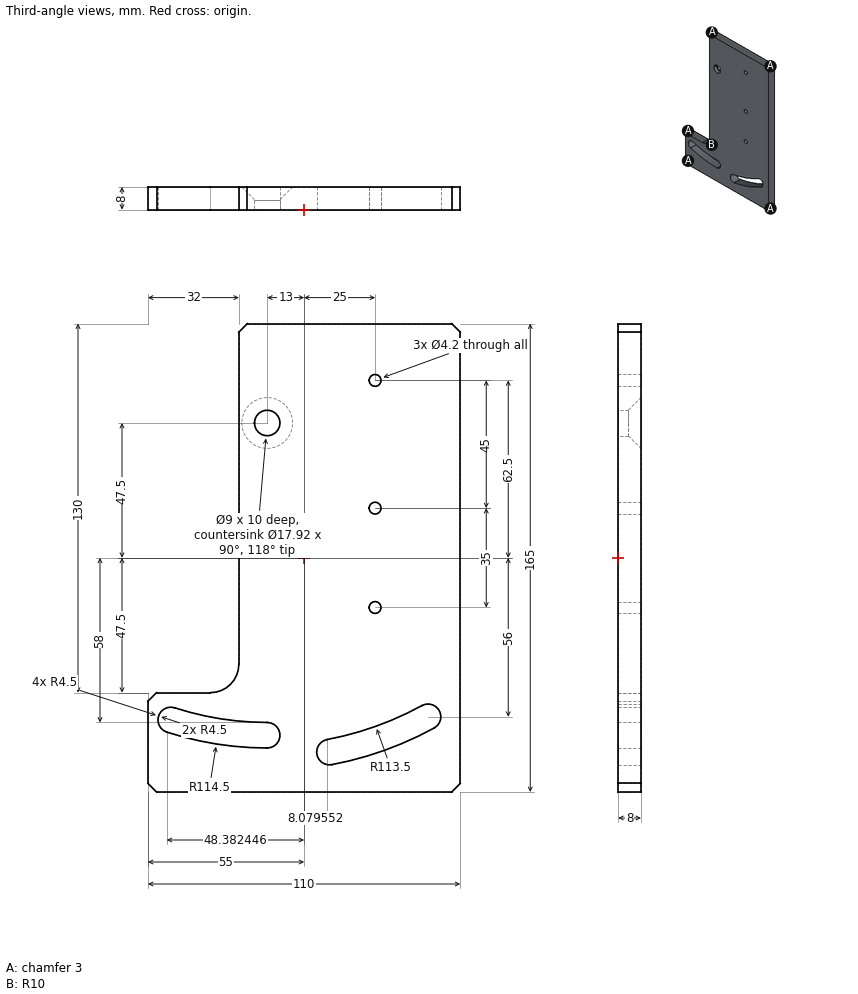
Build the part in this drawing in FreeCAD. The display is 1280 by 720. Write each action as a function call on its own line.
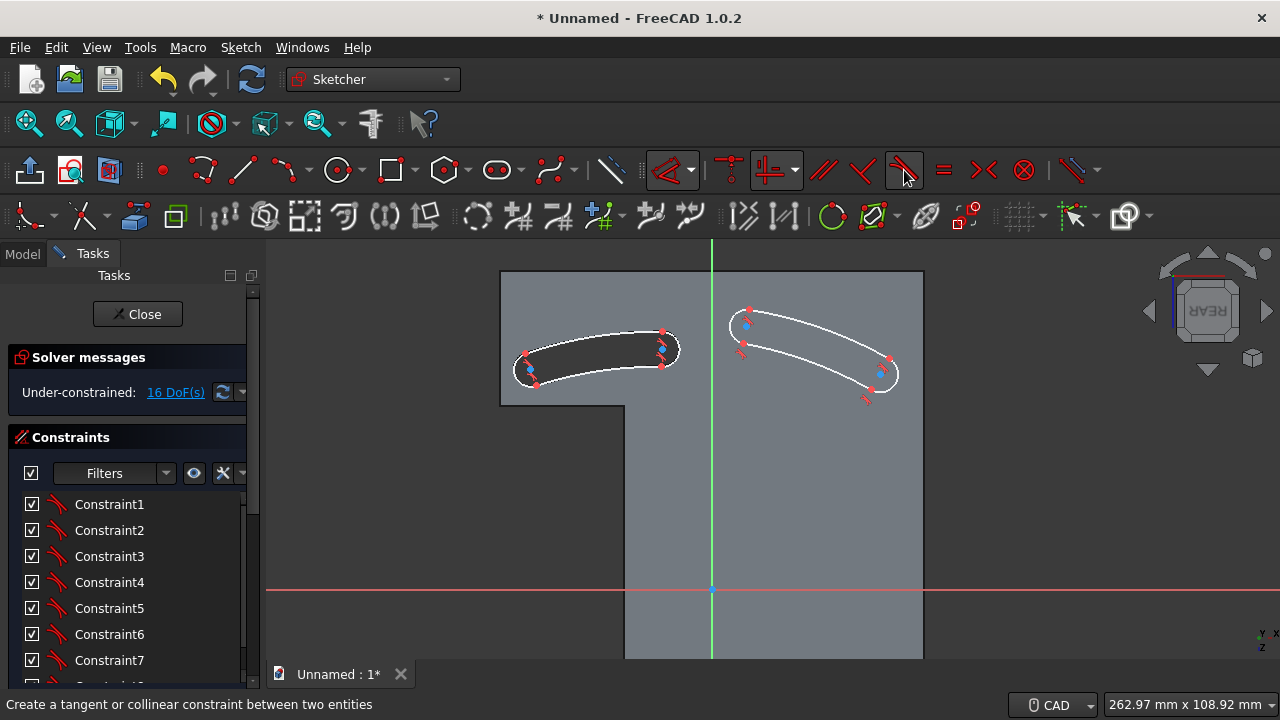
click(621, 333)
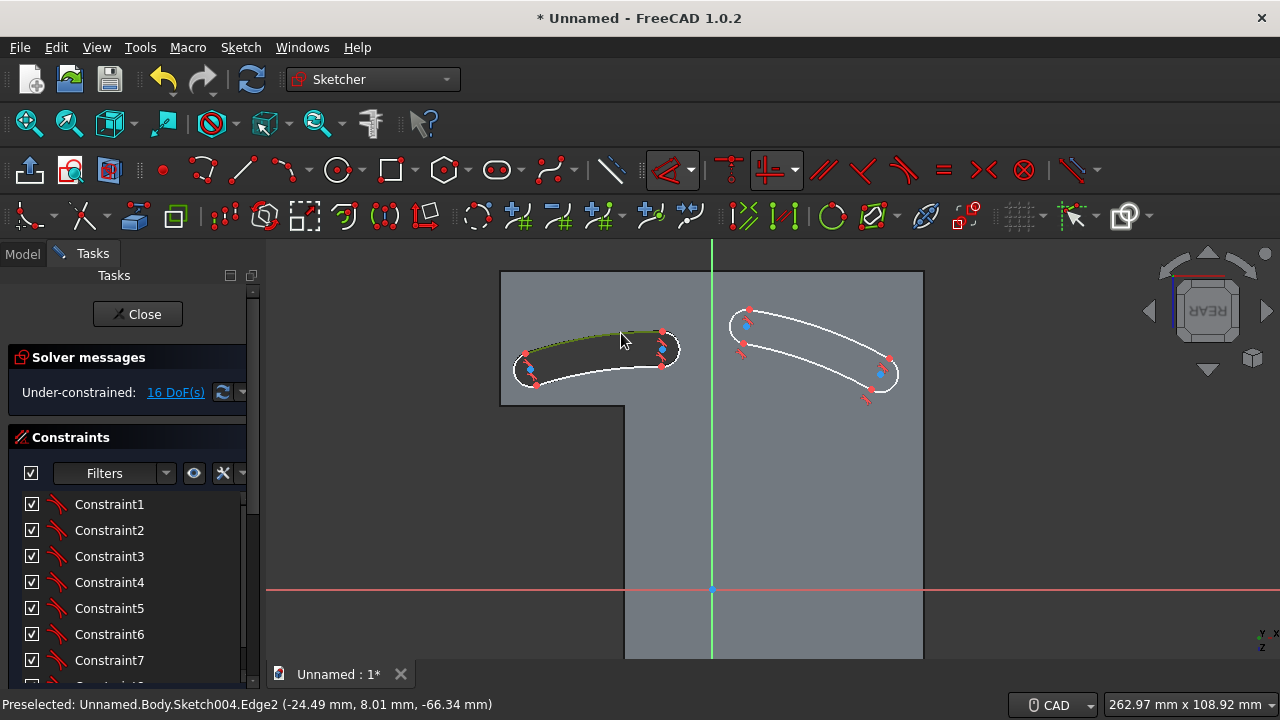
click(624, 368)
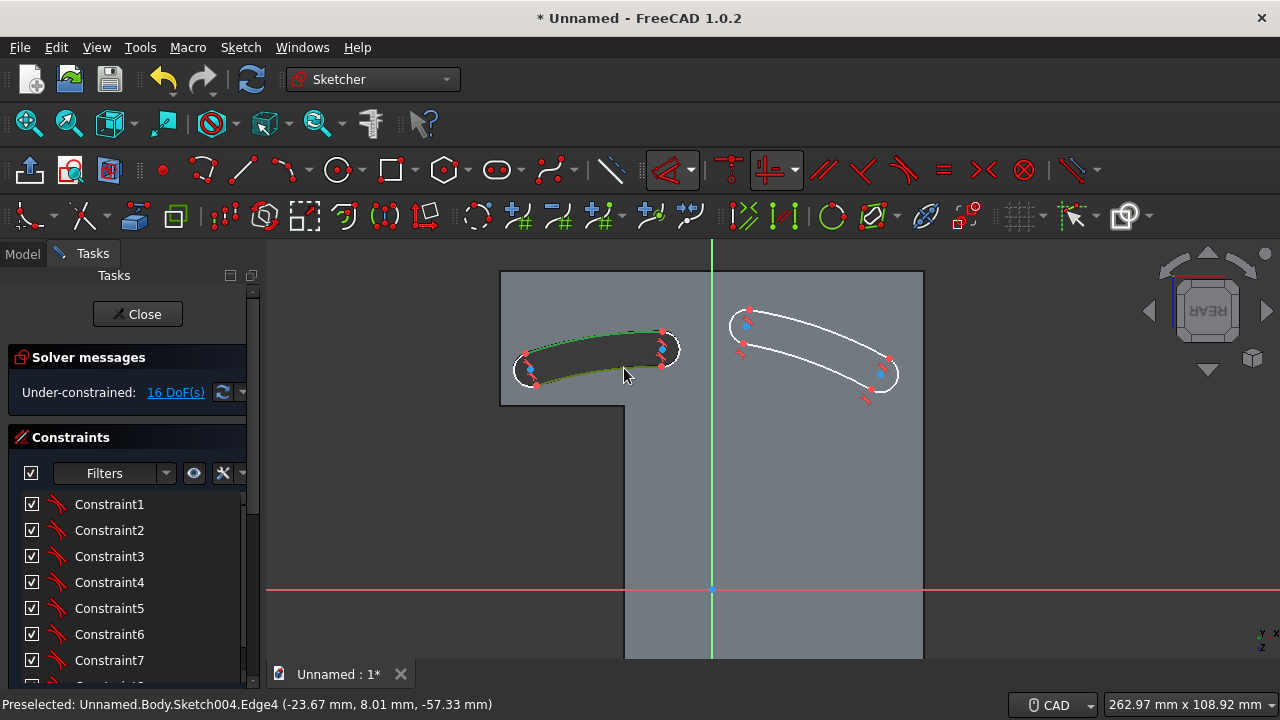
click(730, 170)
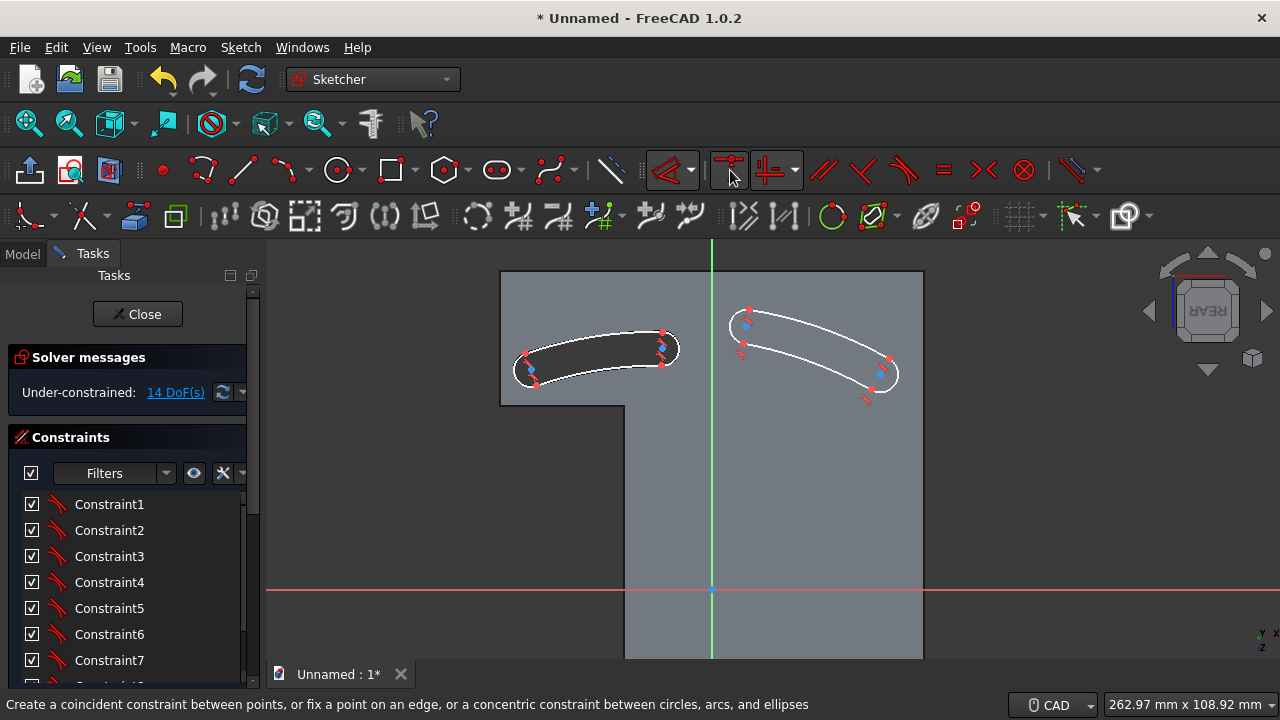
click(621, 333)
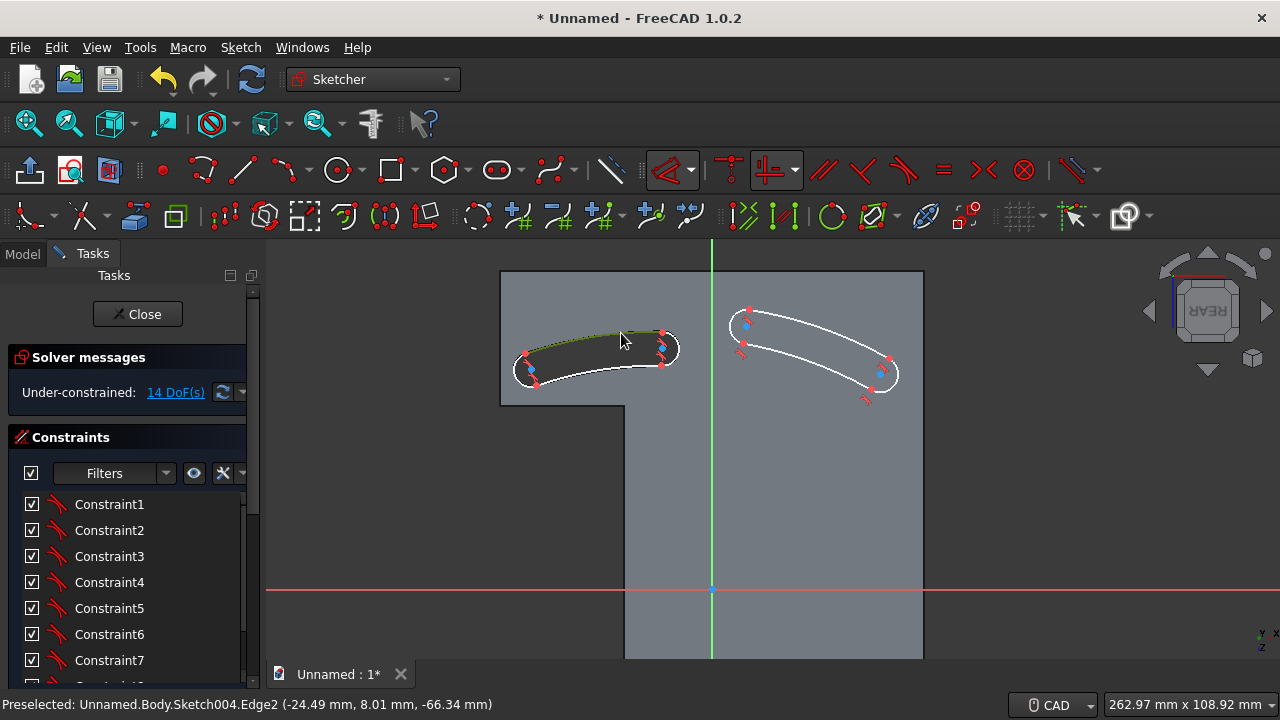
click(835, 372)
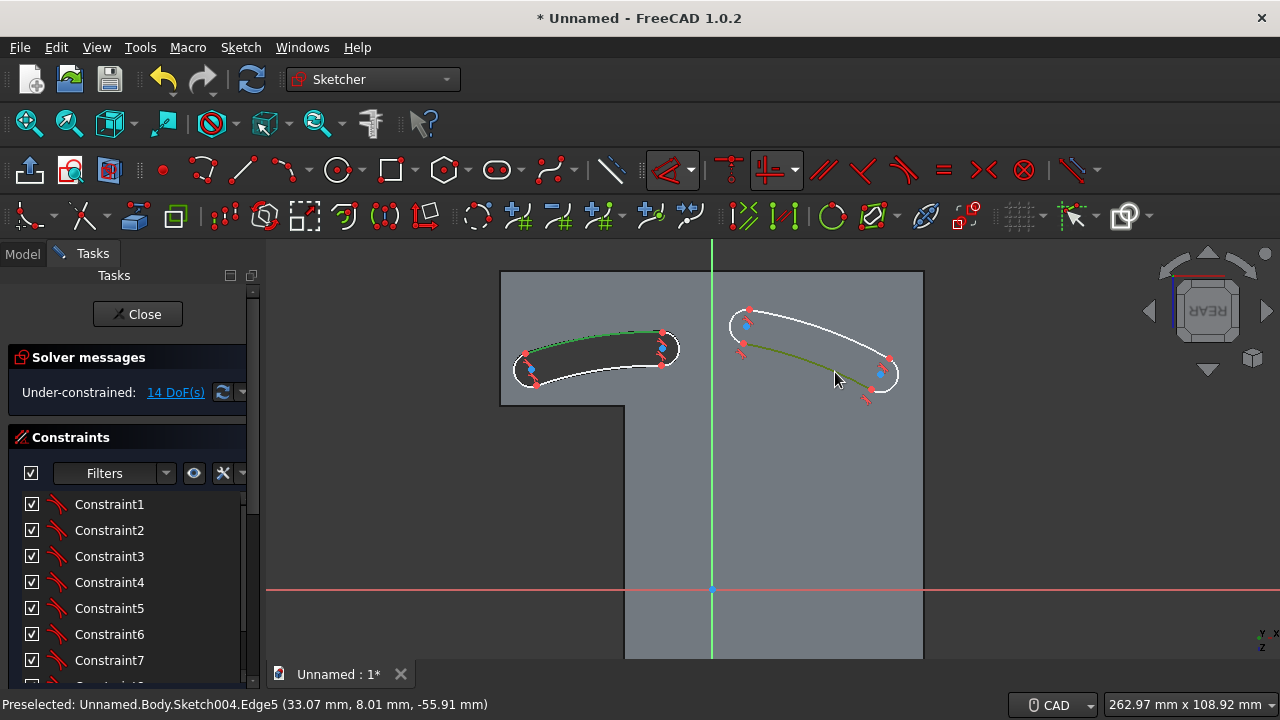
click(730, 170)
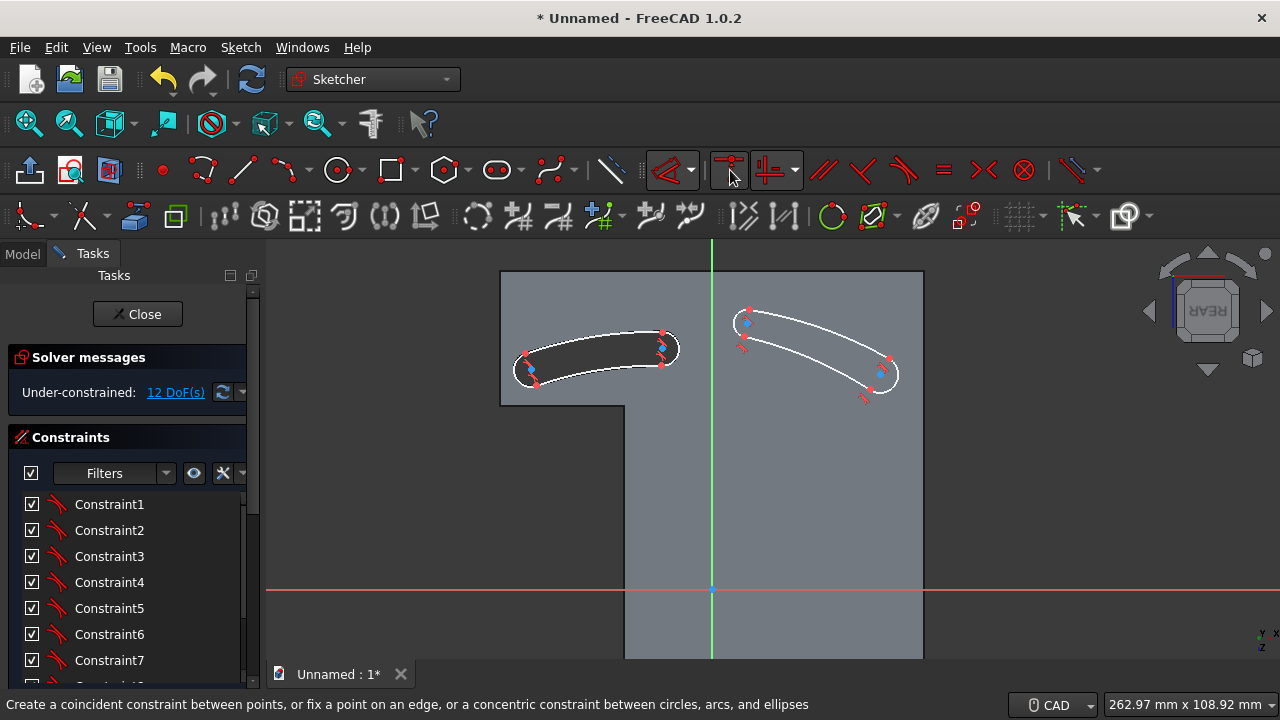
click(621, 333)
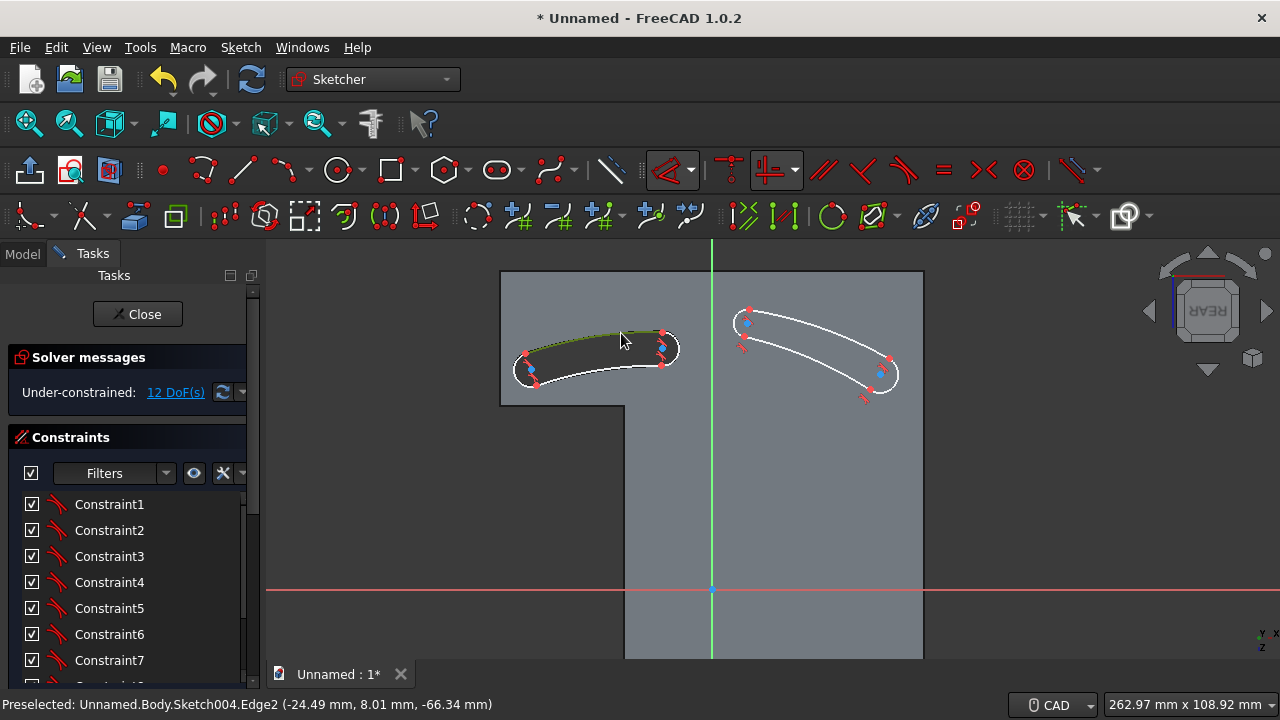
click(849, 339)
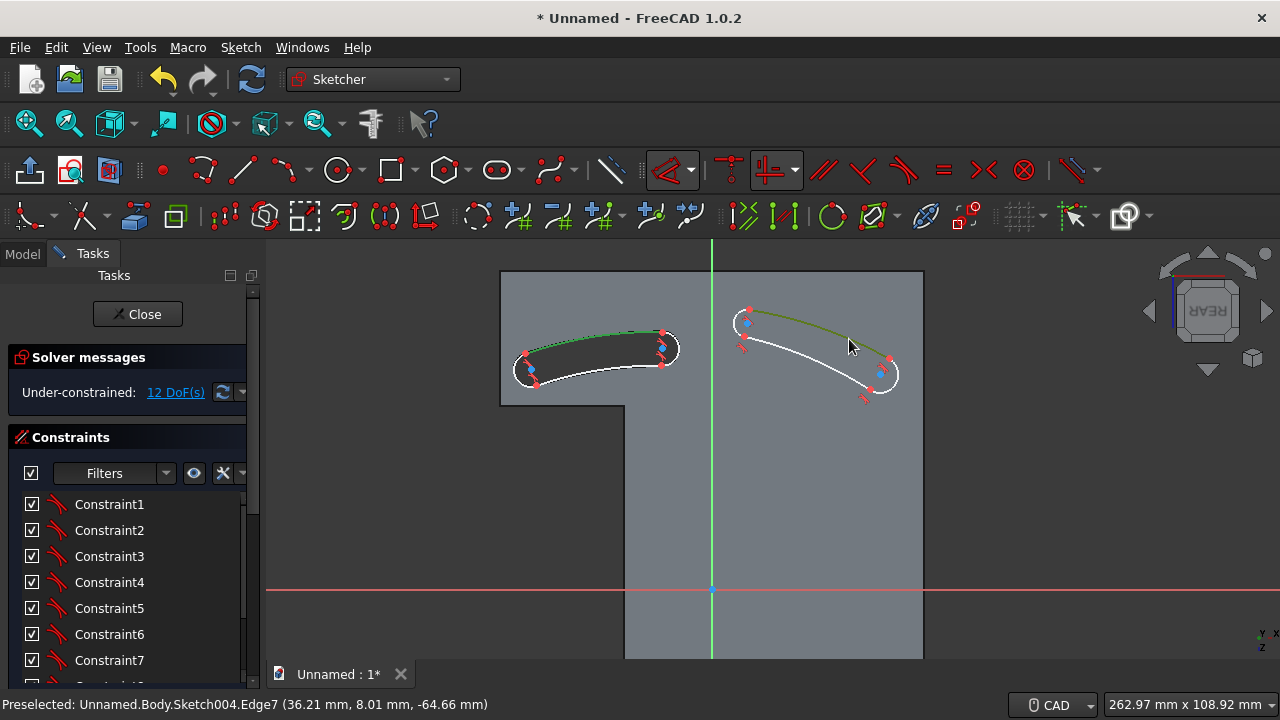
click(730, 170)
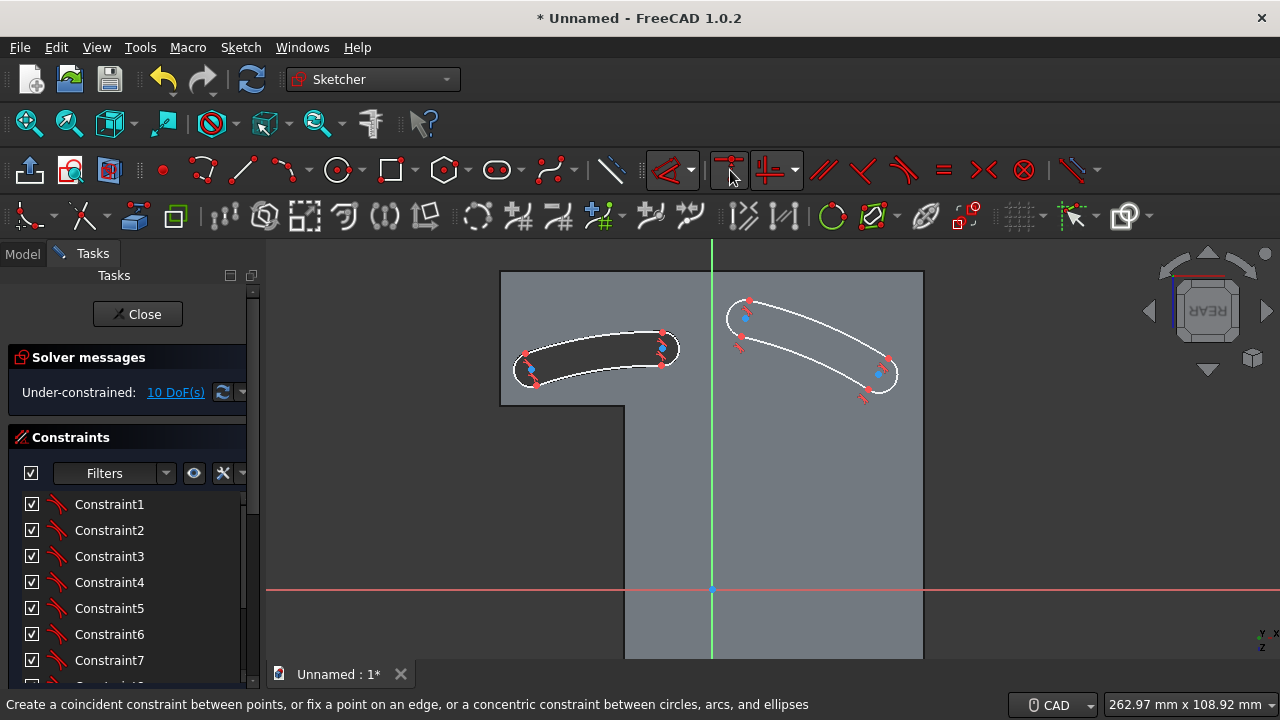
click(676, 359)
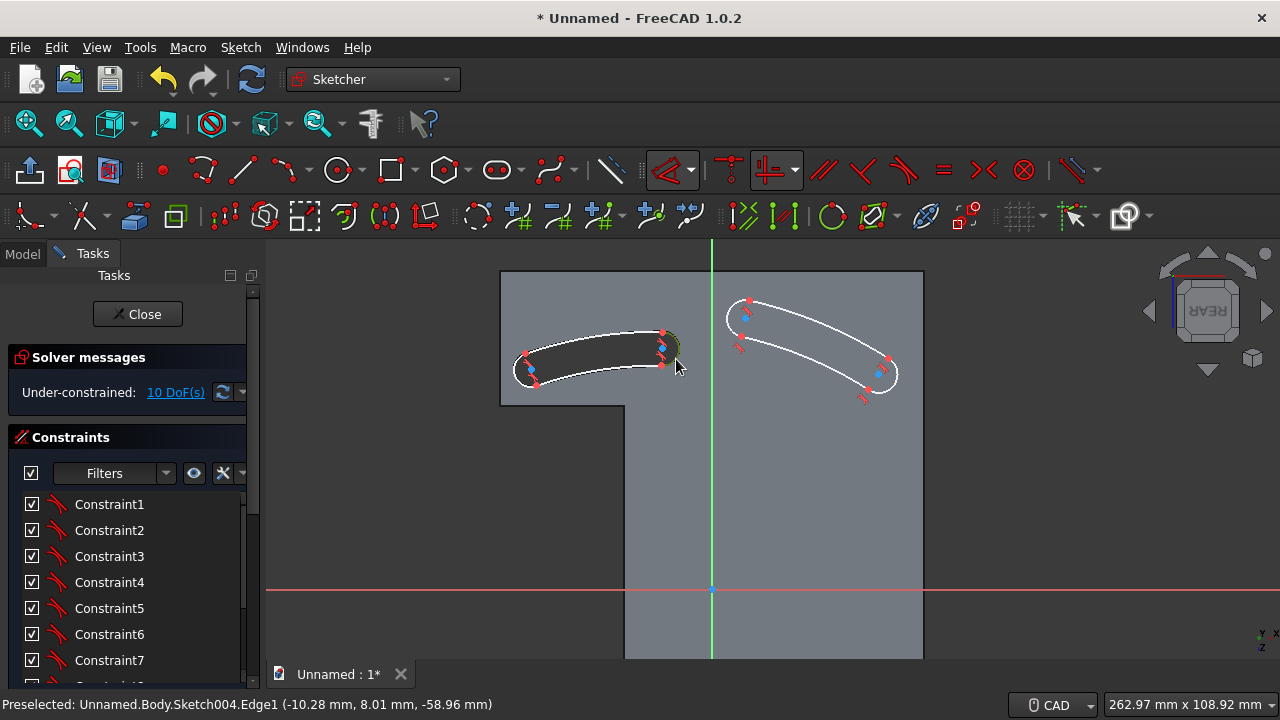
click(886, 392)